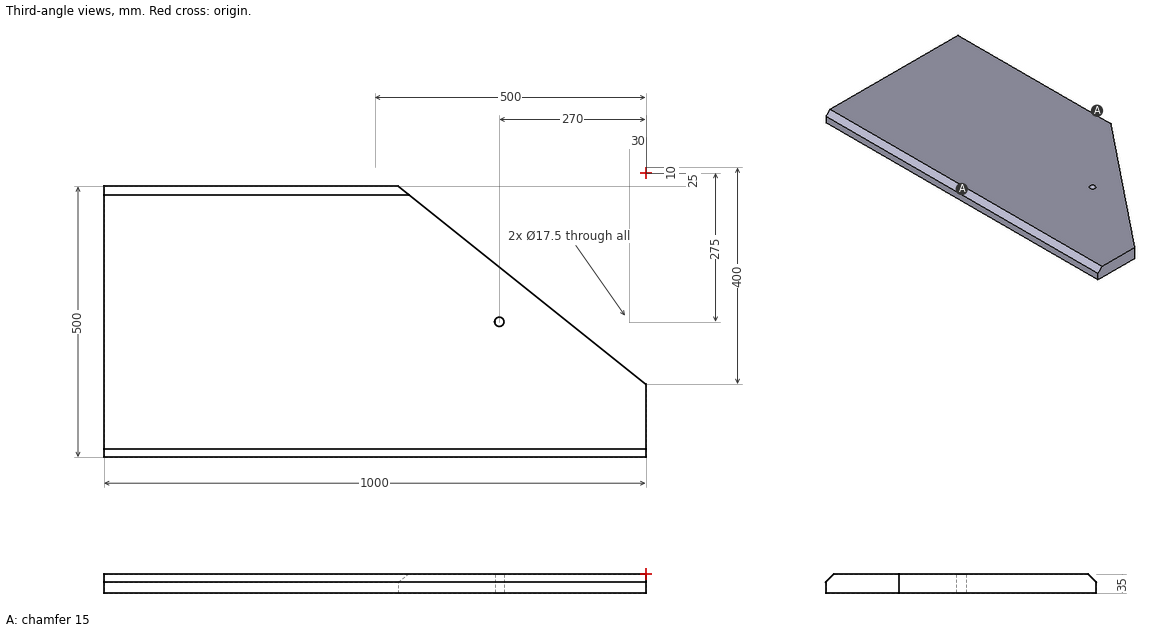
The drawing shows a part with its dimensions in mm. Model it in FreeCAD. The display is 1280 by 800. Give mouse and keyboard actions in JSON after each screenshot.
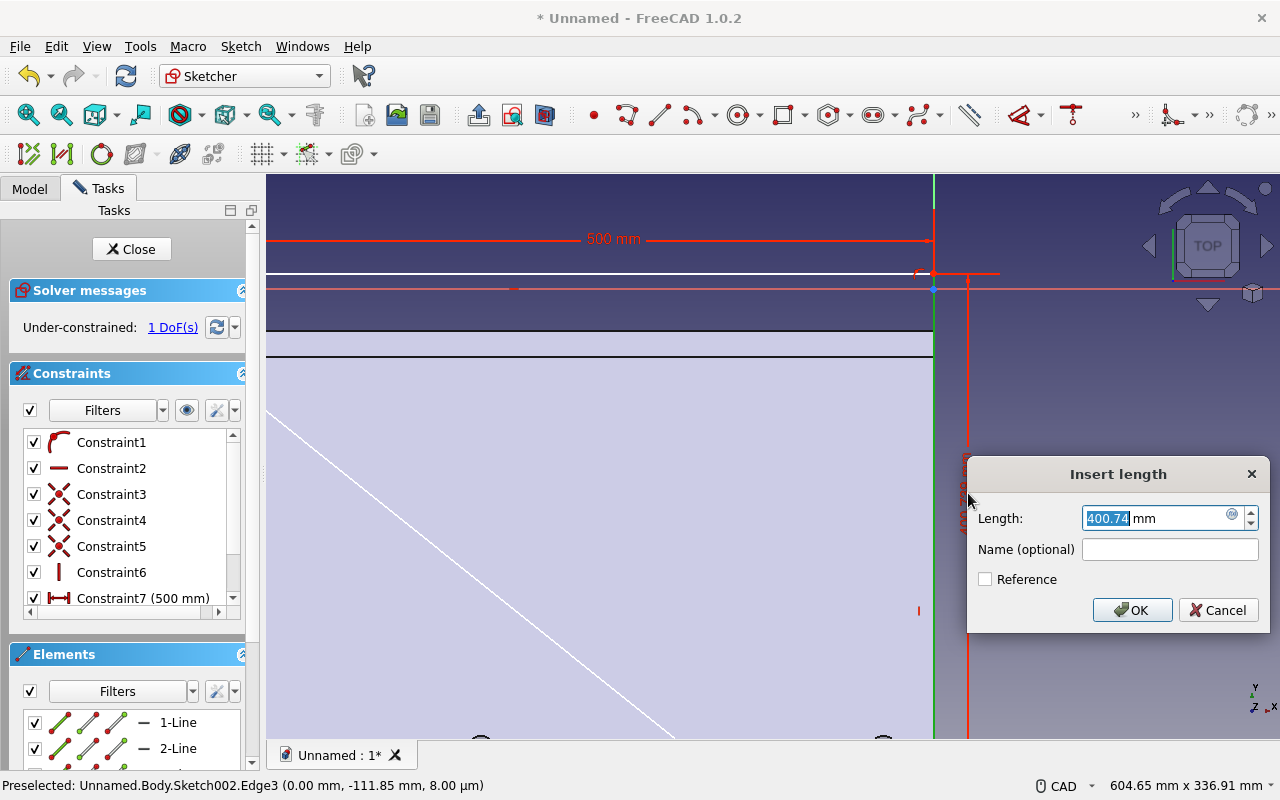
{"action": "type", "text": "400"}
{"action": "key", "text": "Return"}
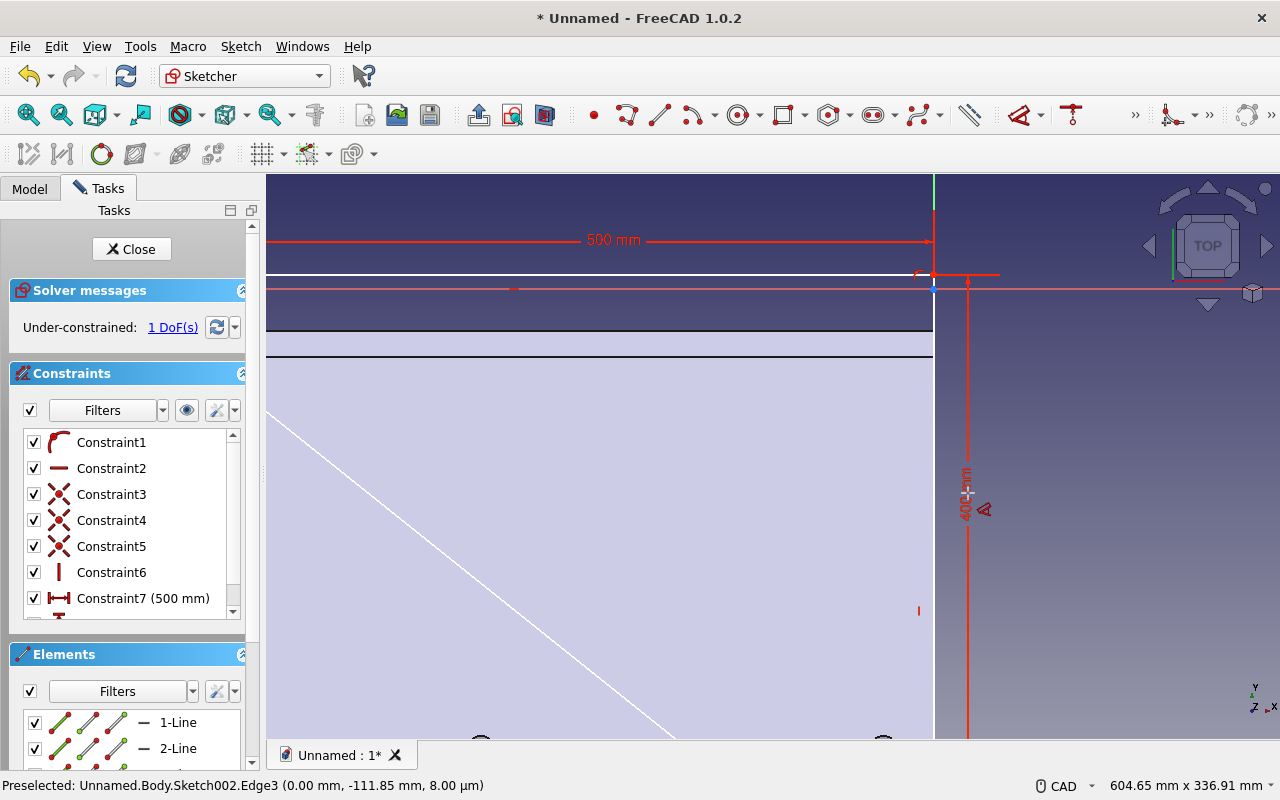
{"action": "scroll", "coordinate": [934, 275], "scroll_direction": "up", "scroll_amount": 5}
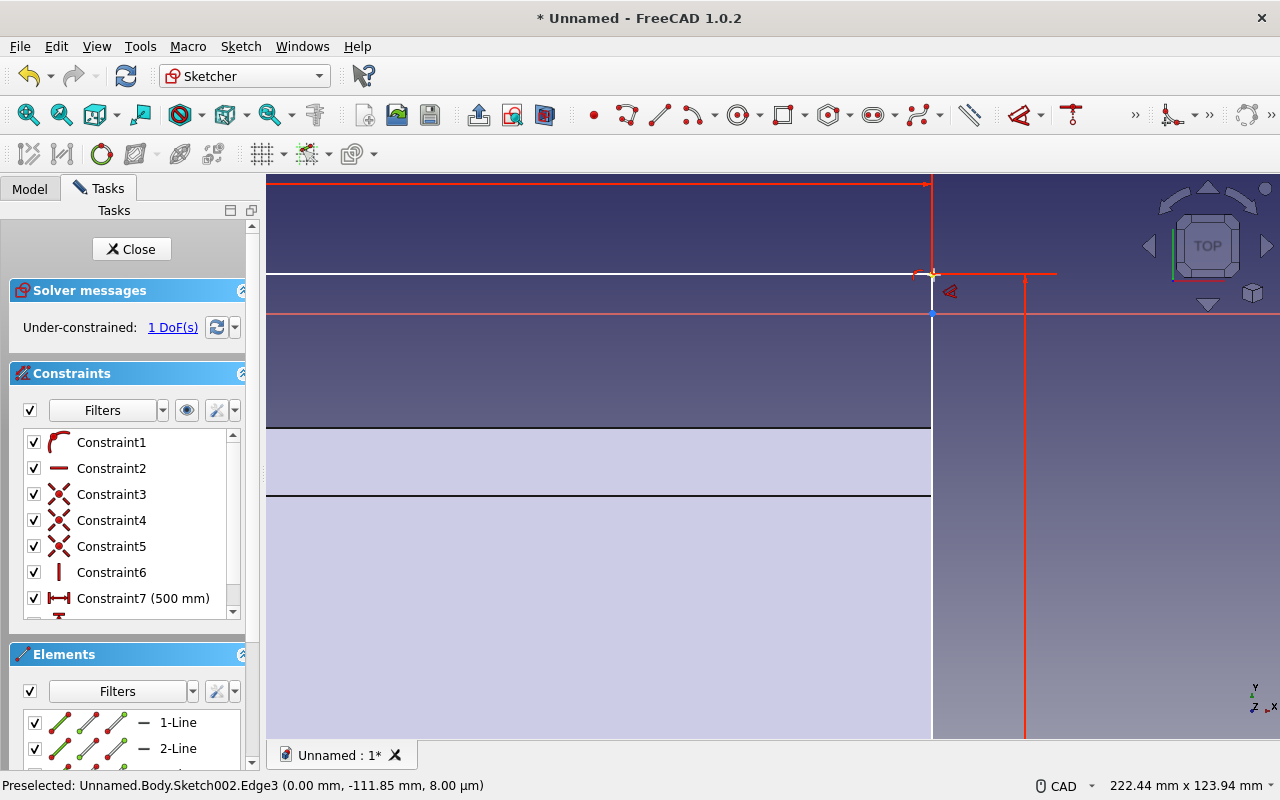
{"action": "left_click", "coordinate": [932, 274]}
{"action": "left_click", "coordinate": [966, 294]}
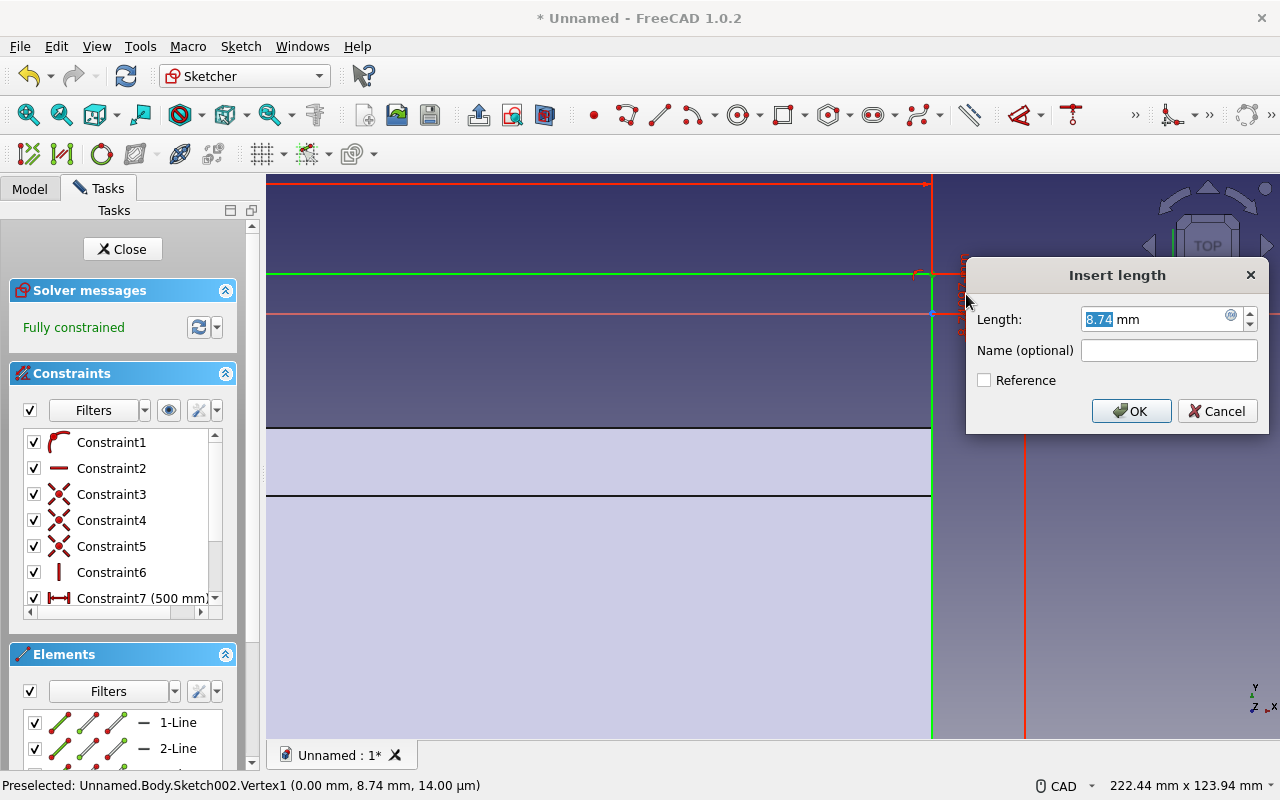
{"action": "type", "text": "10"}
{"action": "key", "text": "Return"}
{"action": "key", "text": "Escape"}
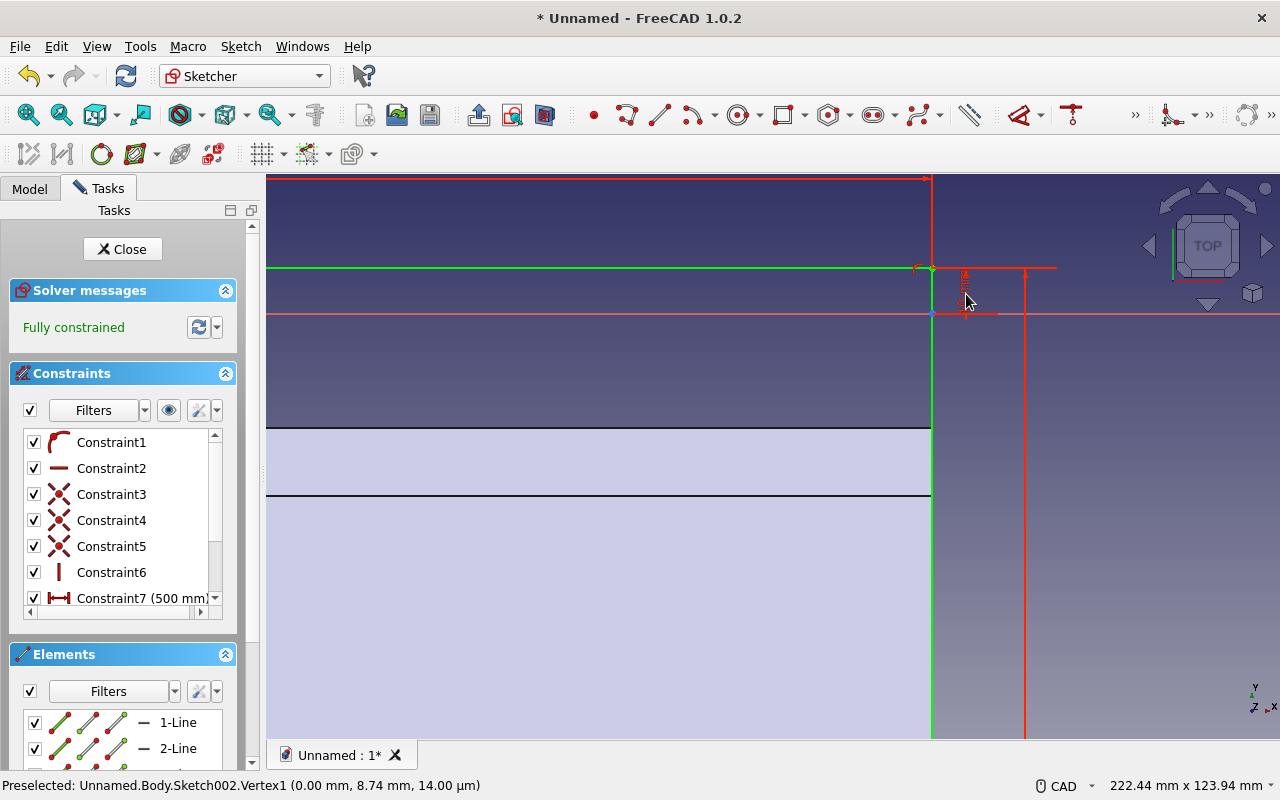
{"action": "left_click", "coordinate": [123, 249]}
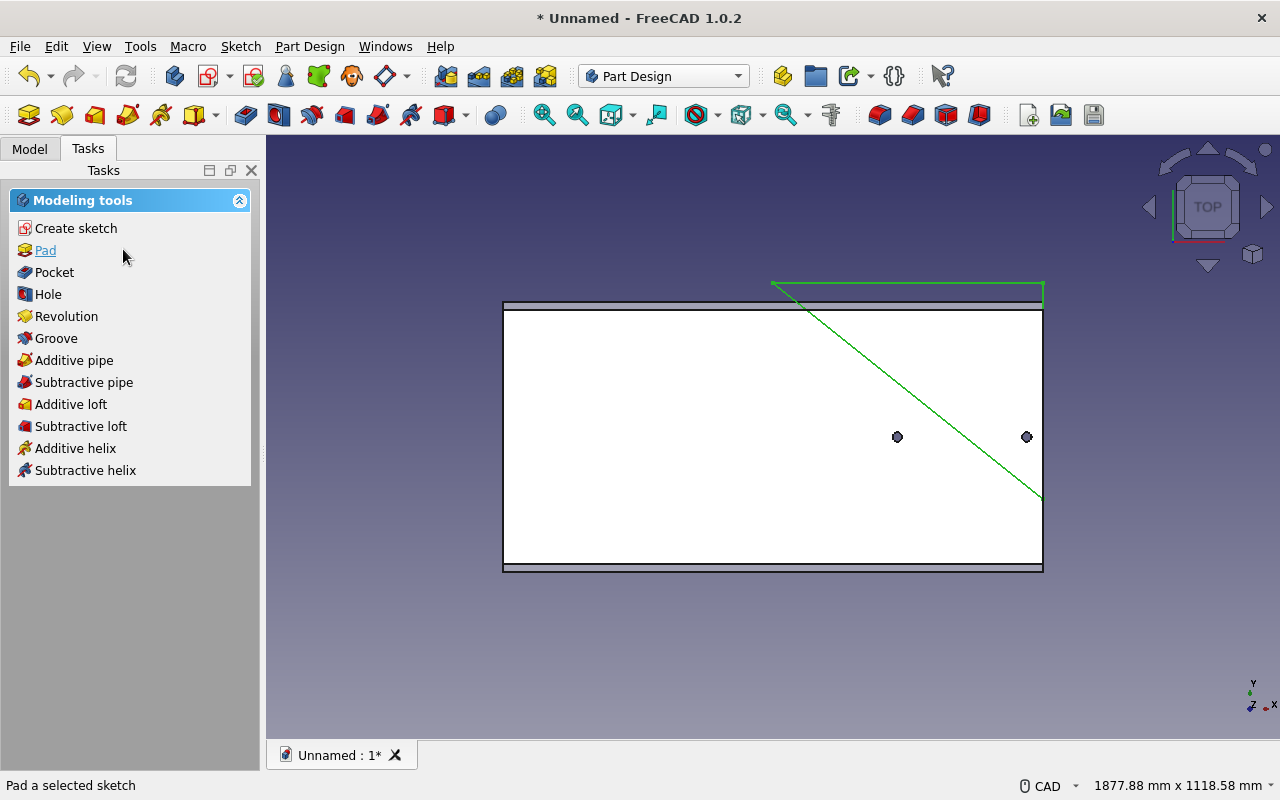
{"action": "left_click", "coordinate": [246, 116]}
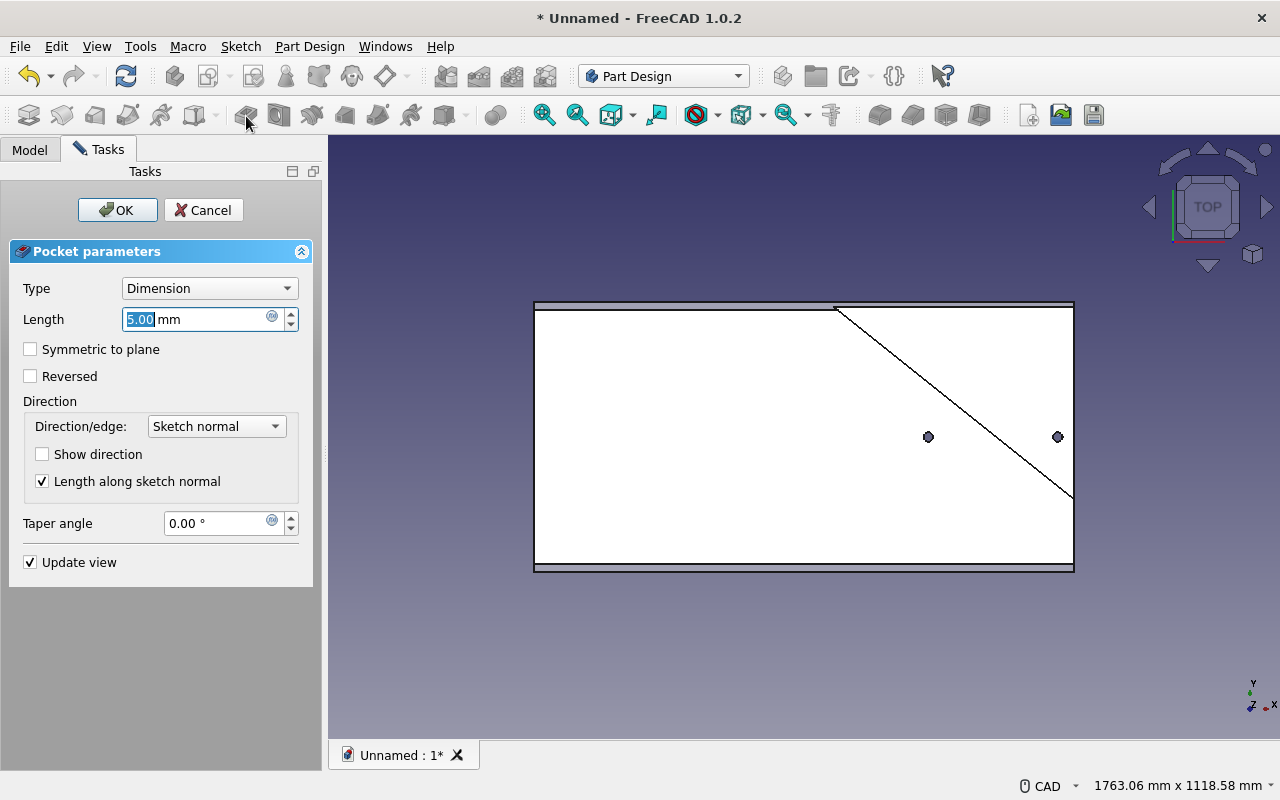
{"action": "left_click", "coordinate": [210, 288]}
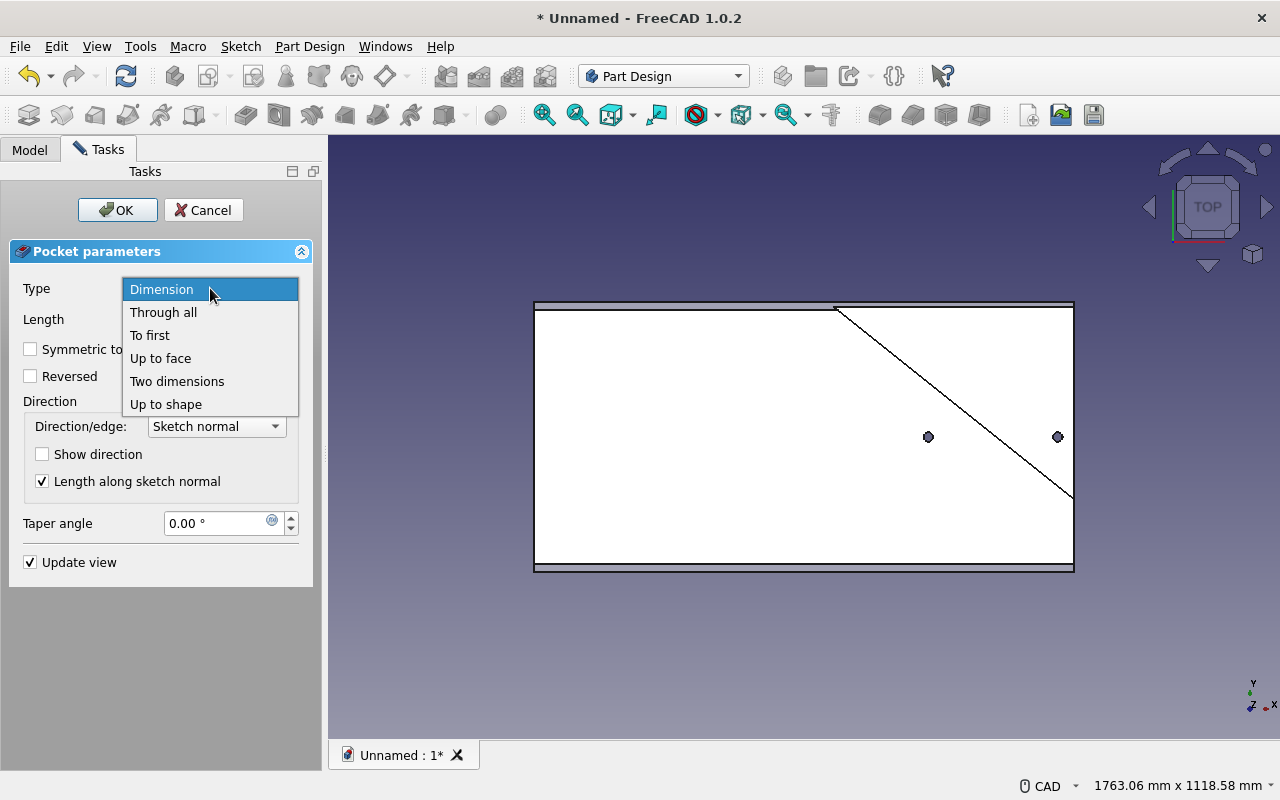
{"action": "left_click", "coordinate": [208, 312]}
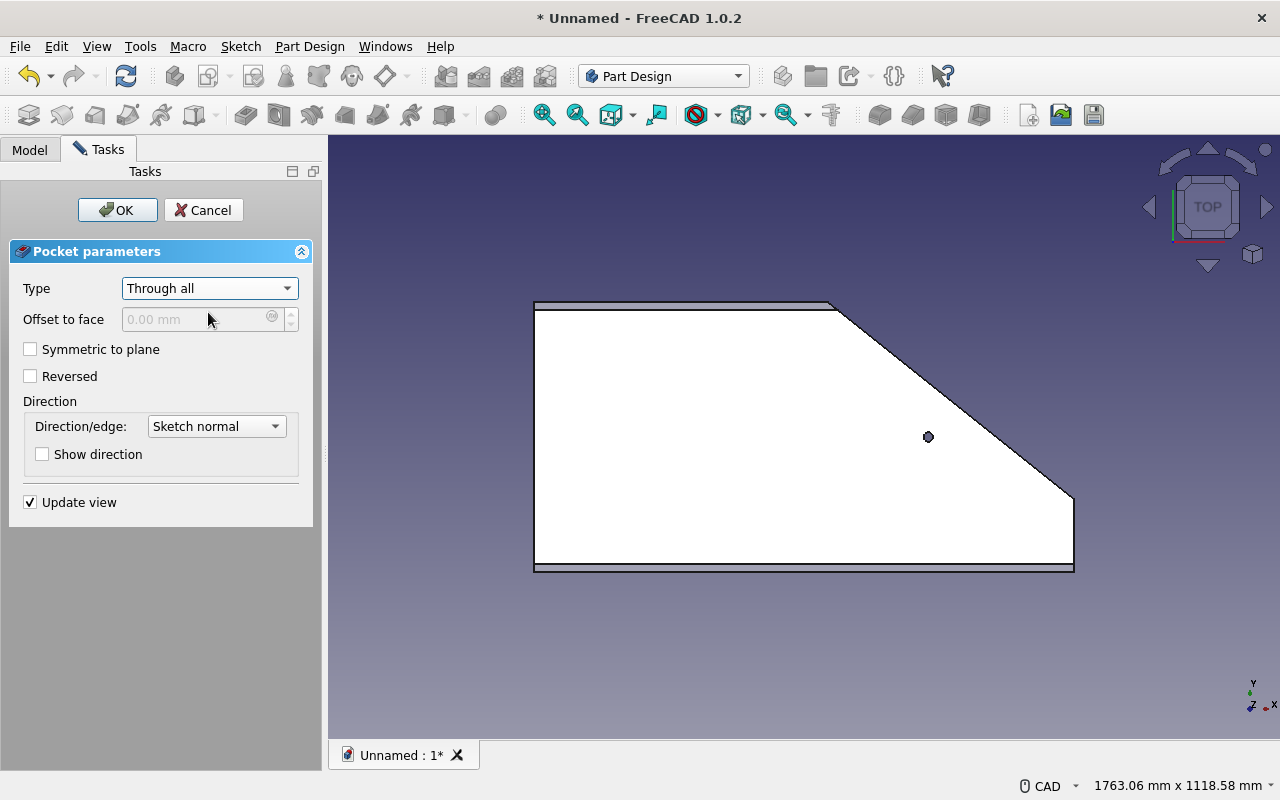
{"action": "left_click", "coordinate": [118, 210]}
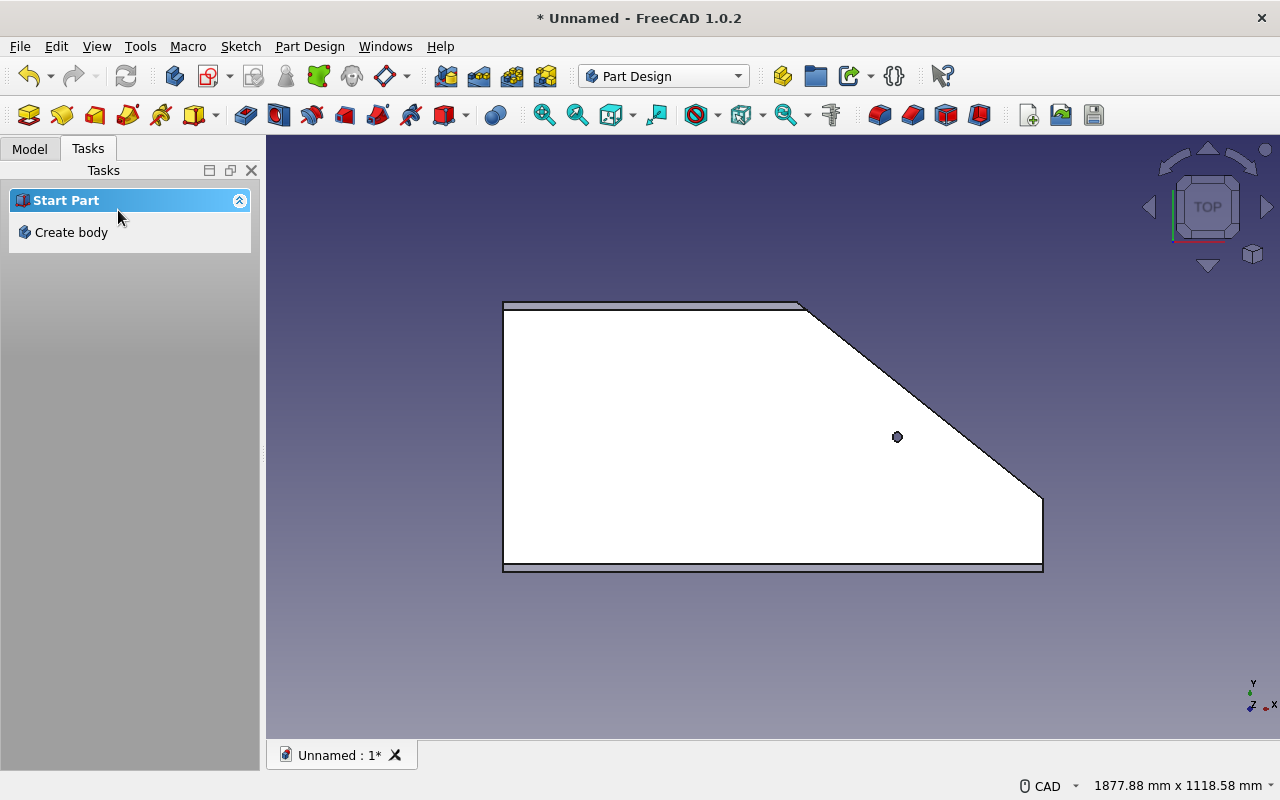
{"action": "key", "text": "0"}